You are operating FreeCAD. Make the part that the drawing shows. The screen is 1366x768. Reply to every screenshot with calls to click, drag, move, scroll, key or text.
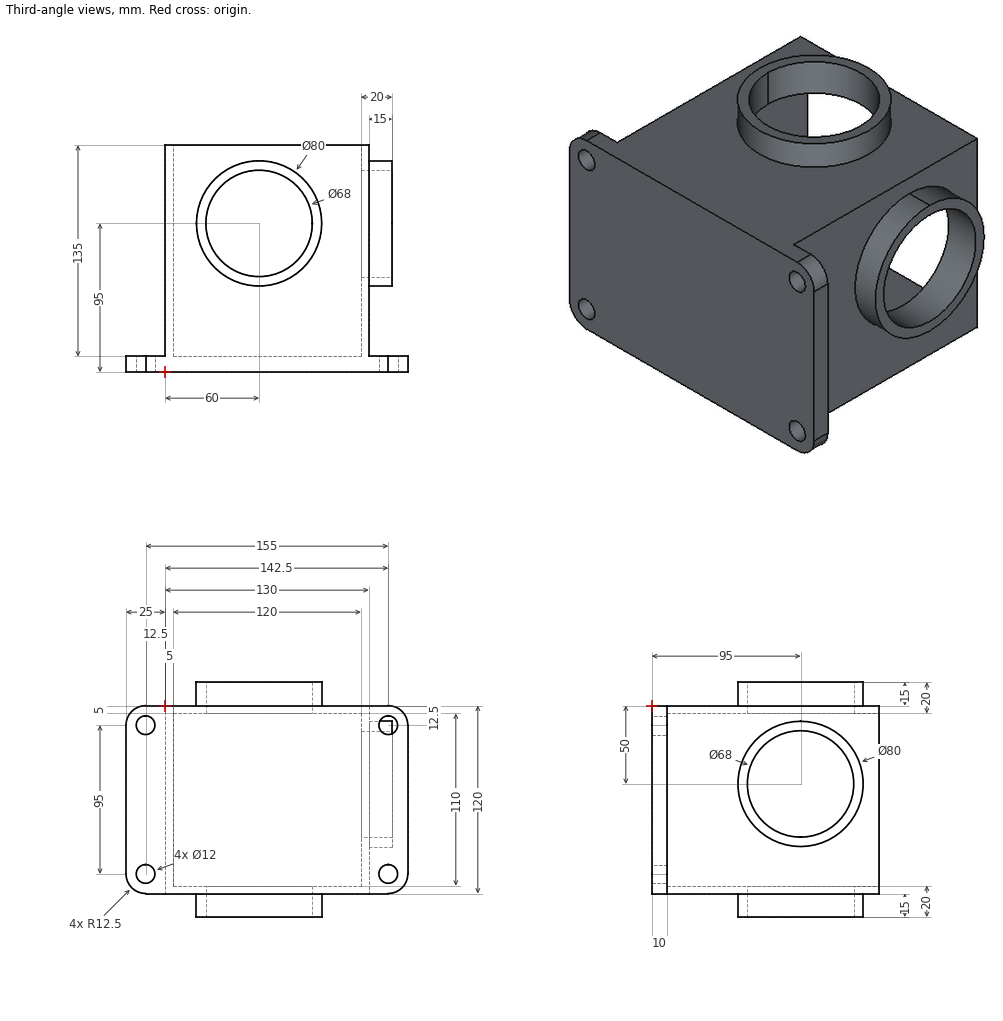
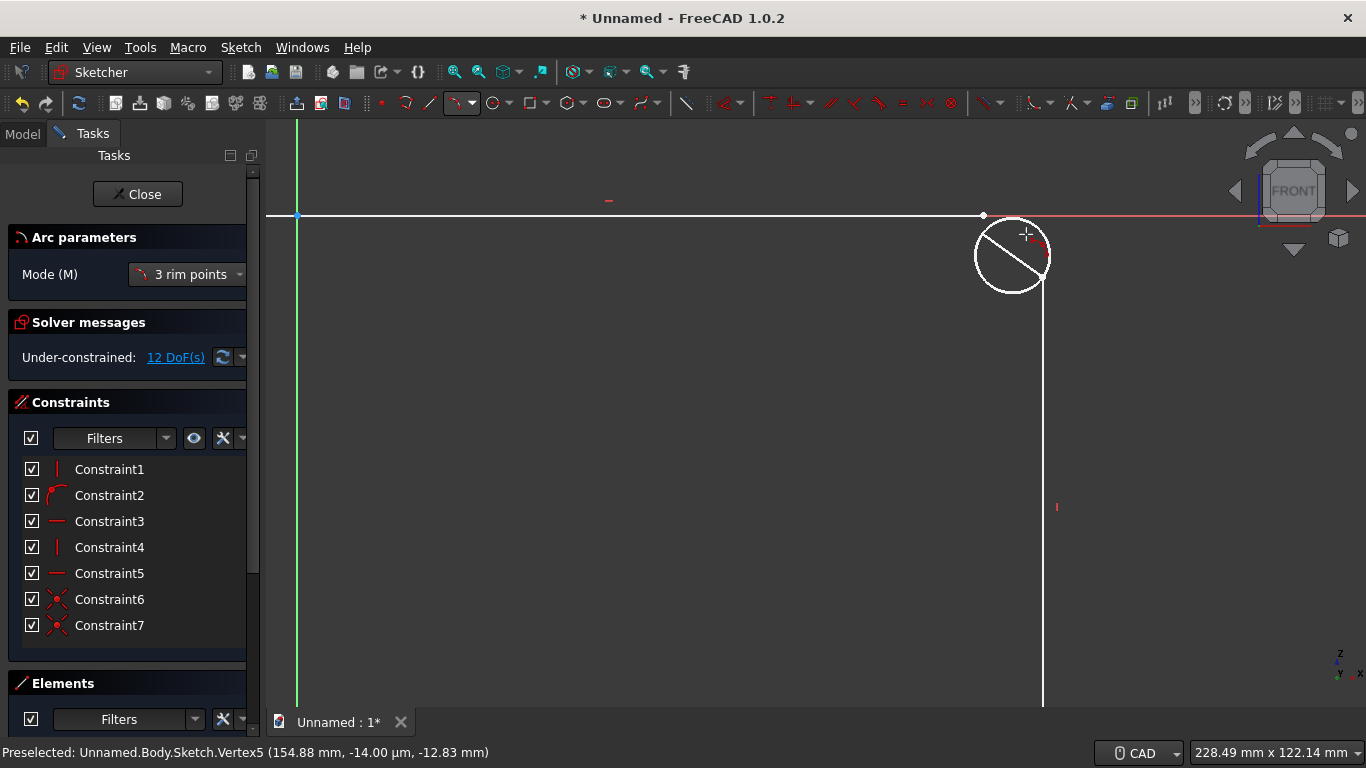
click(1026, 233)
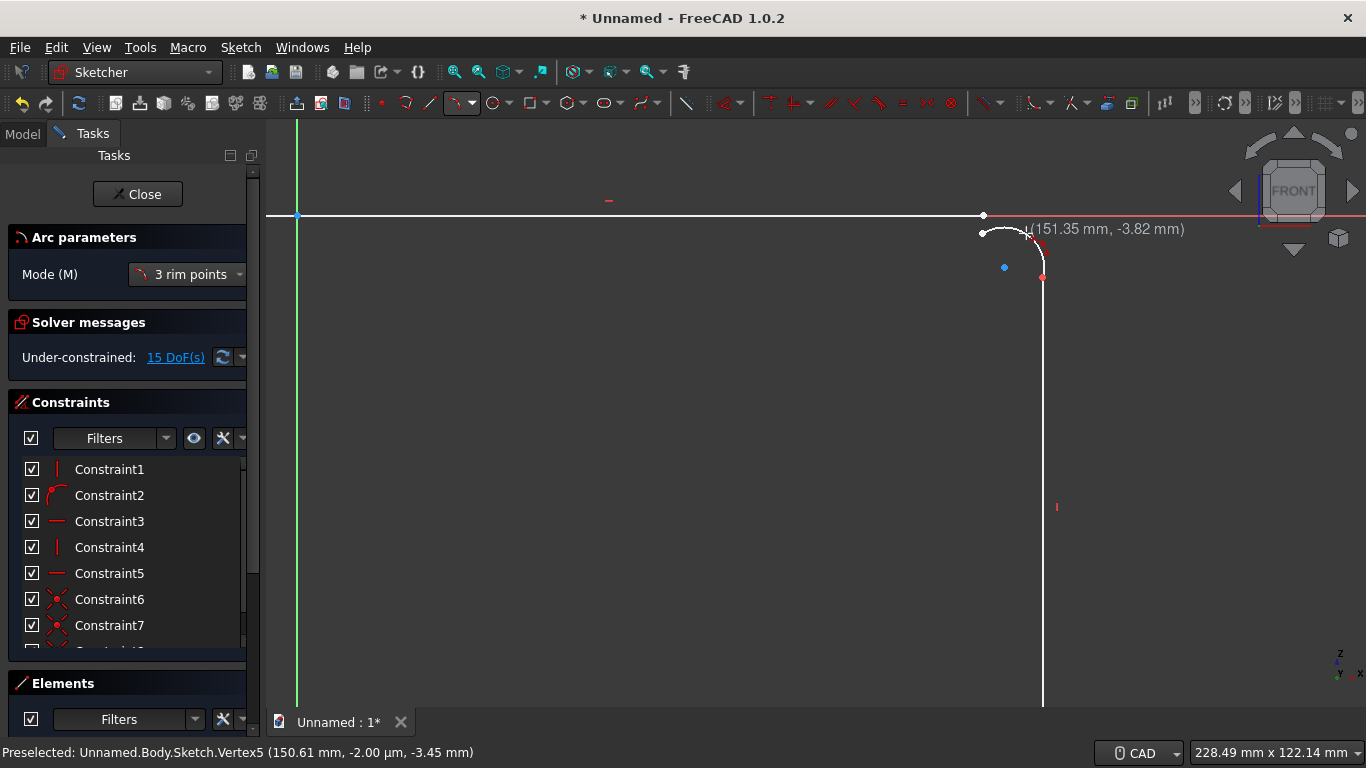
scroll(1026, 227, down, 2)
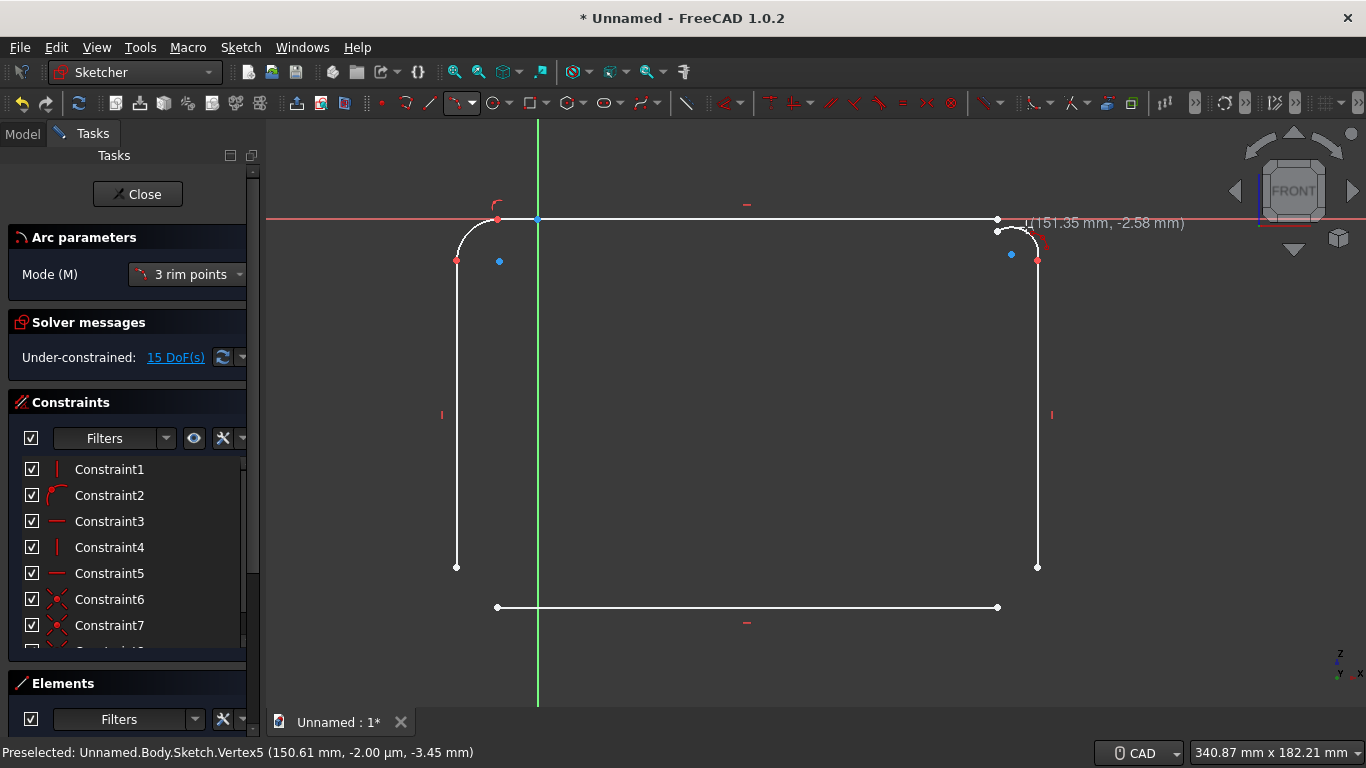
click(1038, 568)
click(997, 608)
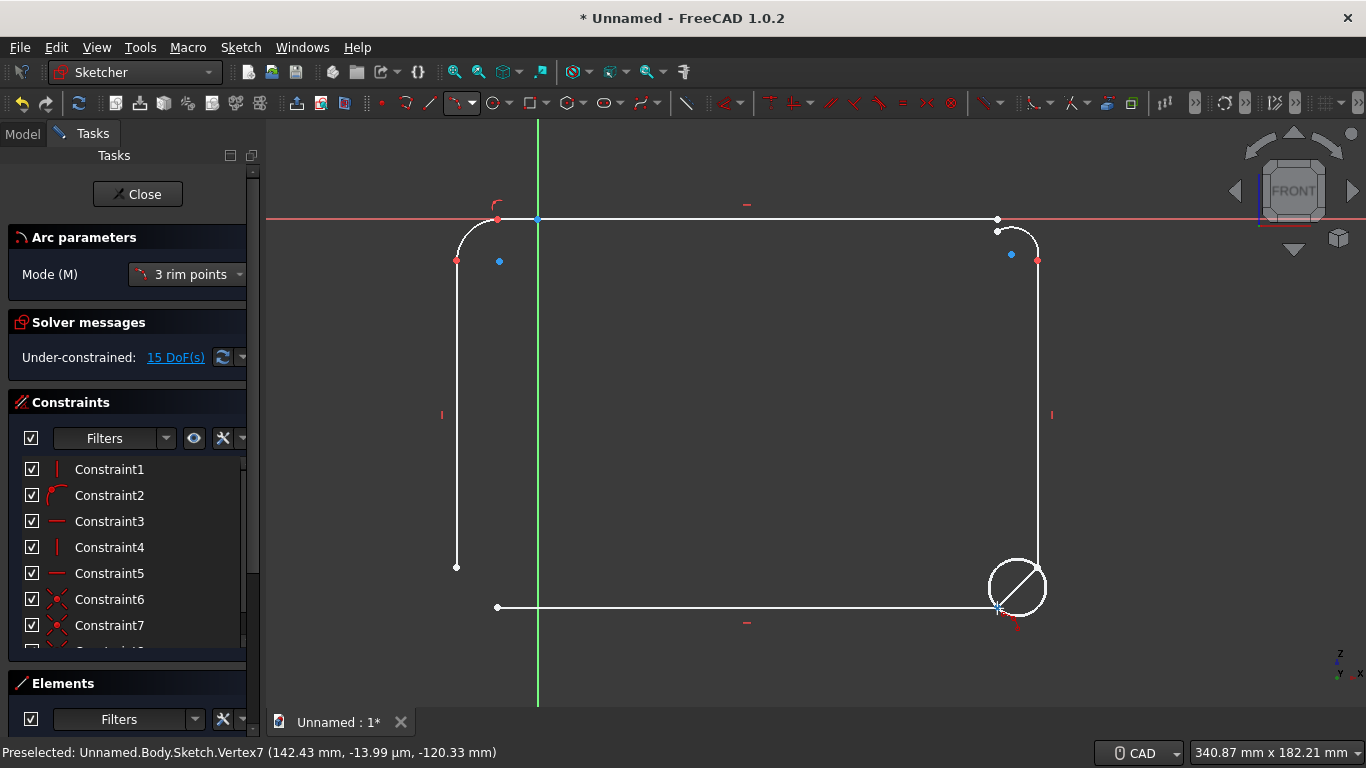
scroll(1026, 595, up, 2)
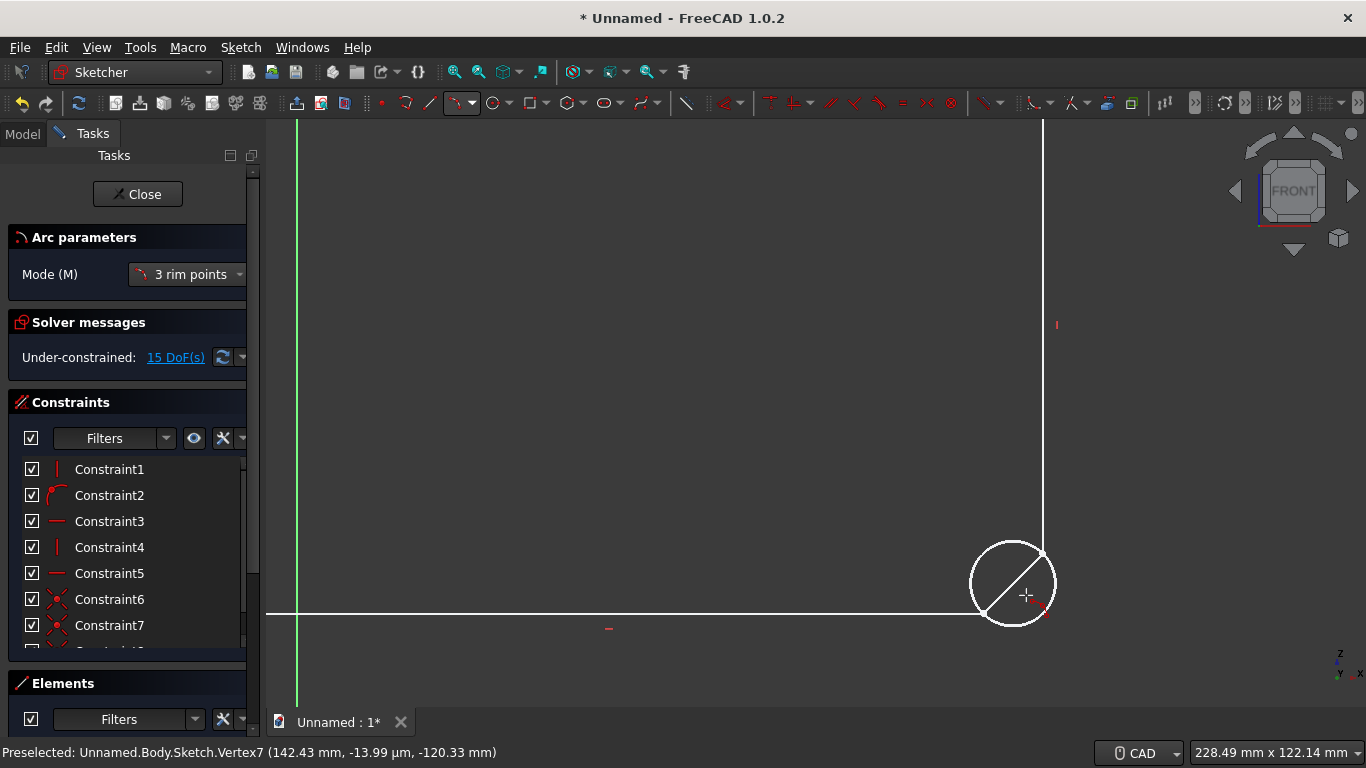
click(1026, 594)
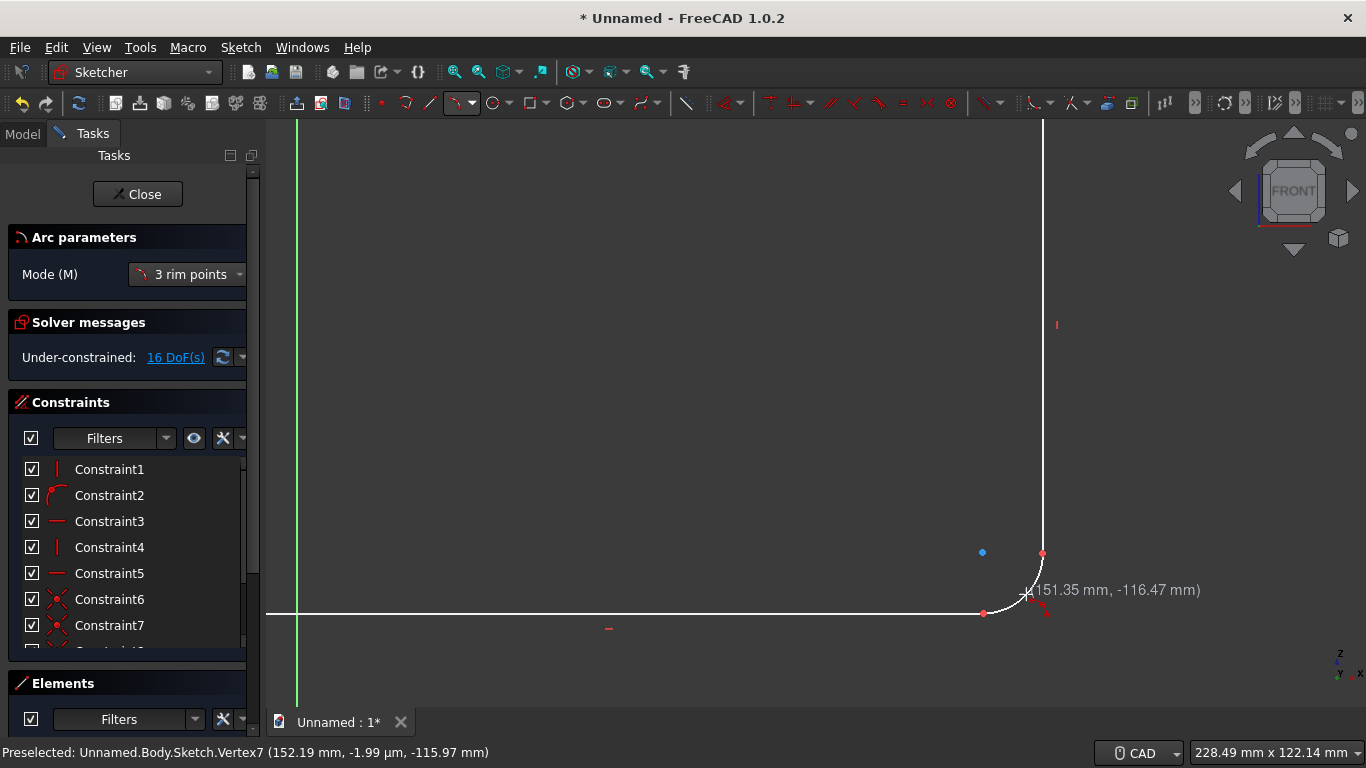
scroll(1026, 596, down, 2)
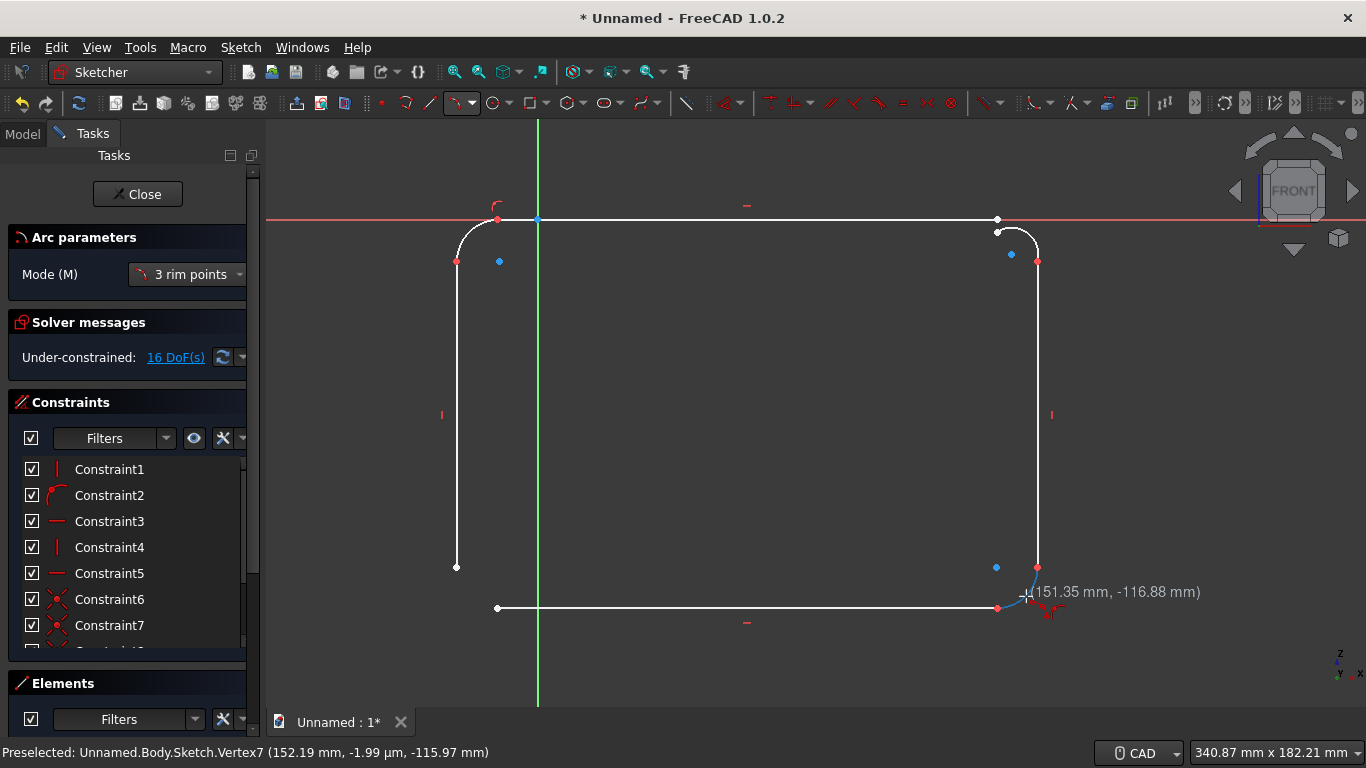
click(497, 608)
click(457, 568)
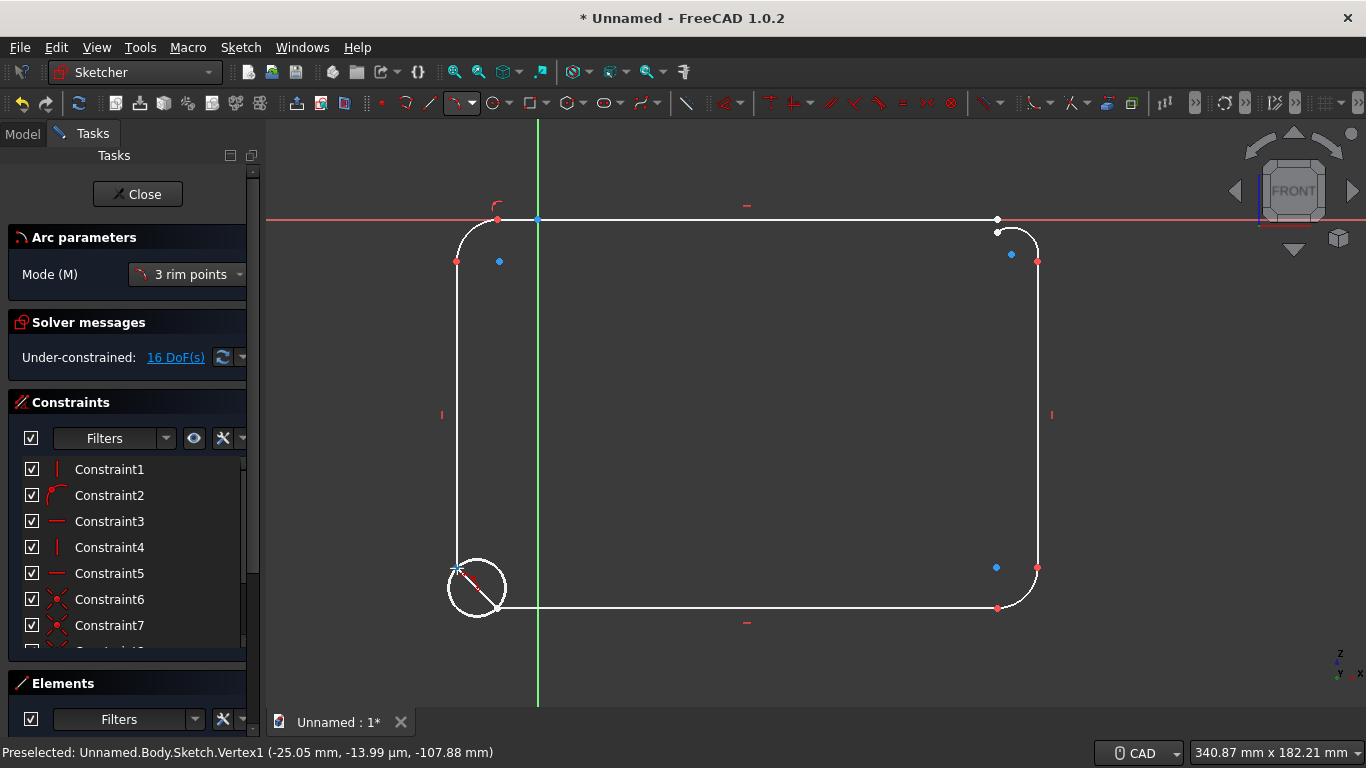
scroll(469, 595, up, 2)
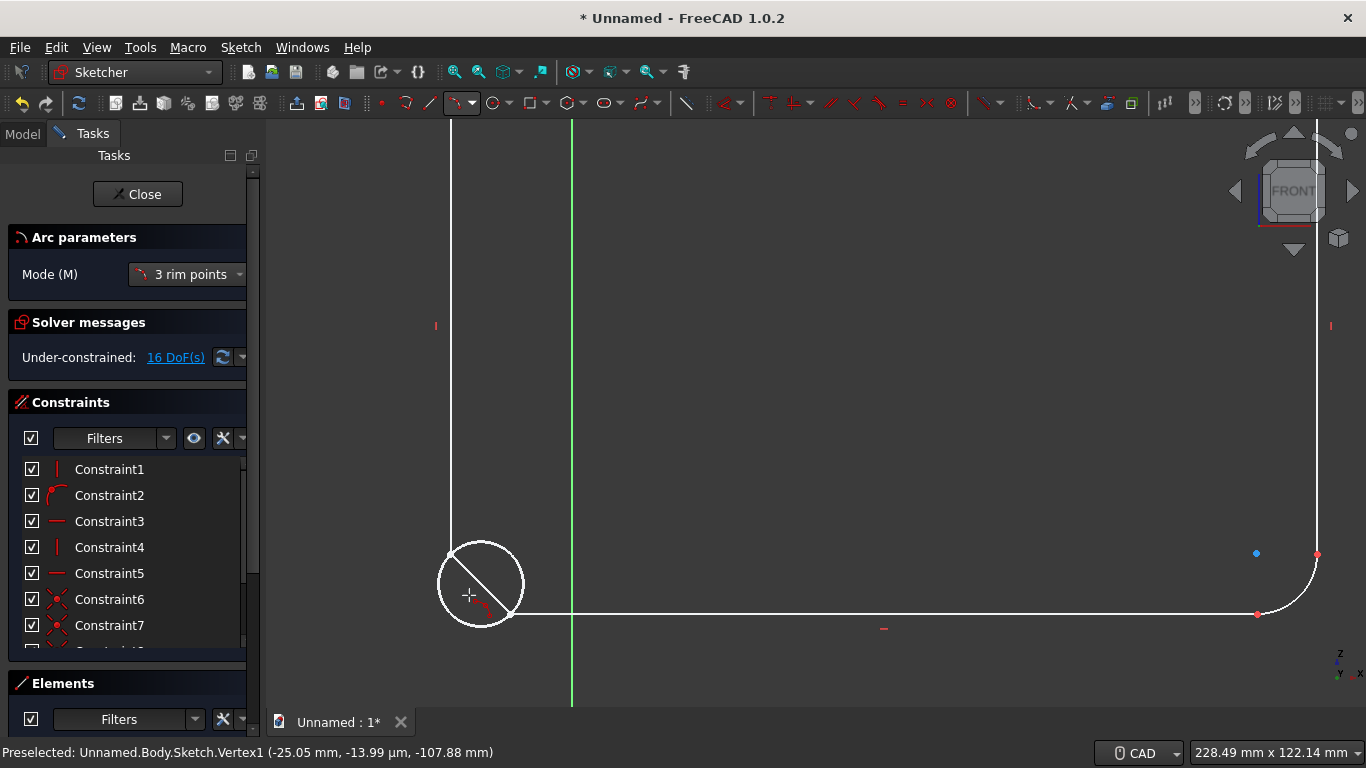
click(469, 595)
key(Escape)